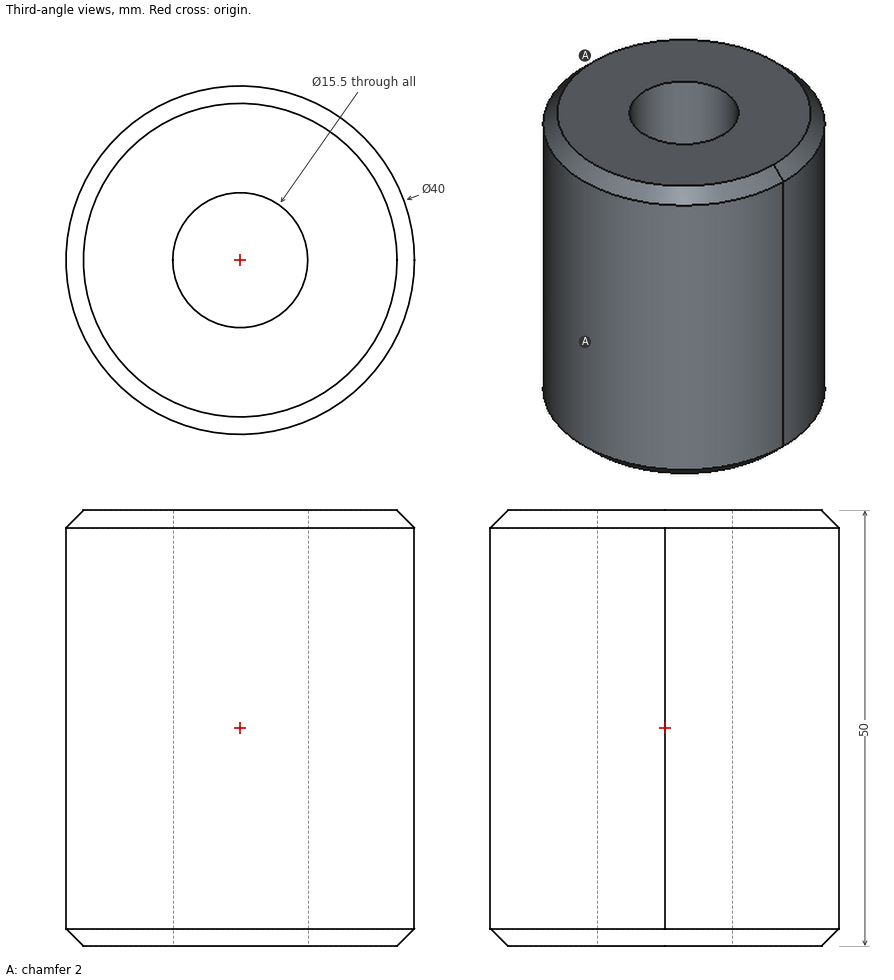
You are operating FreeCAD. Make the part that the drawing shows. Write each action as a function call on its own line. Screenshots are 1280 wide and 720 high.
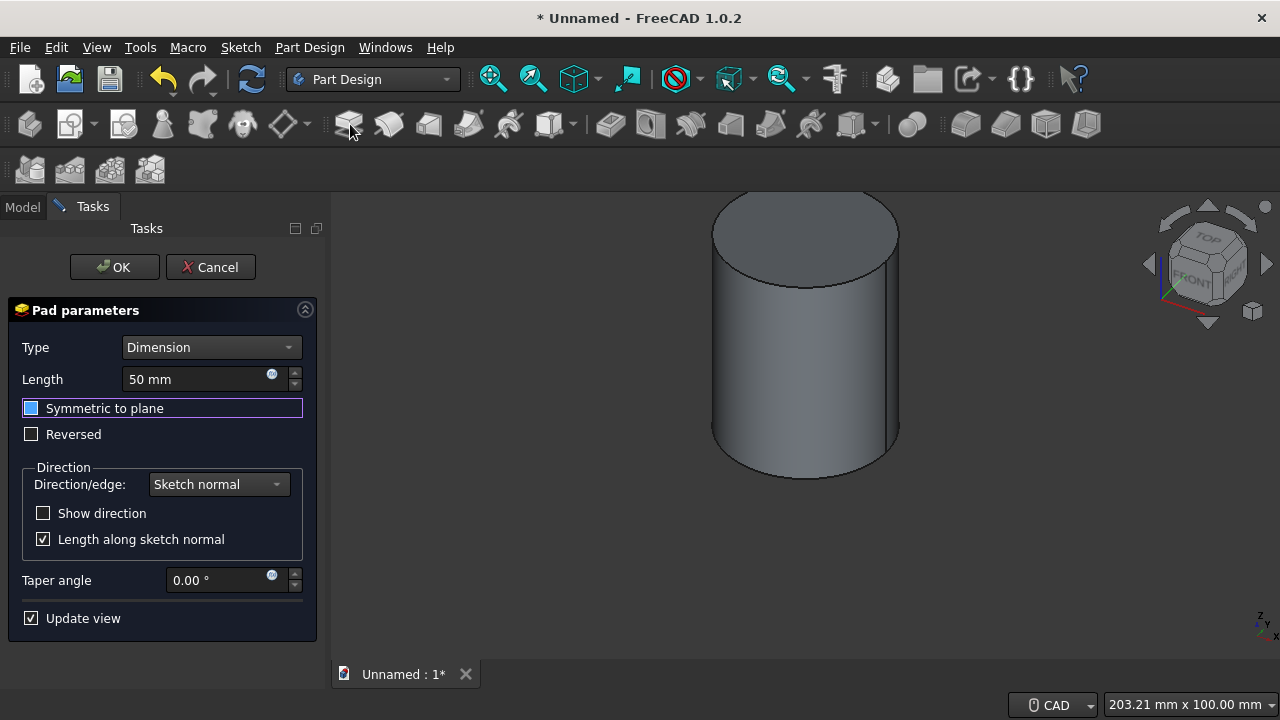
click(30, 408)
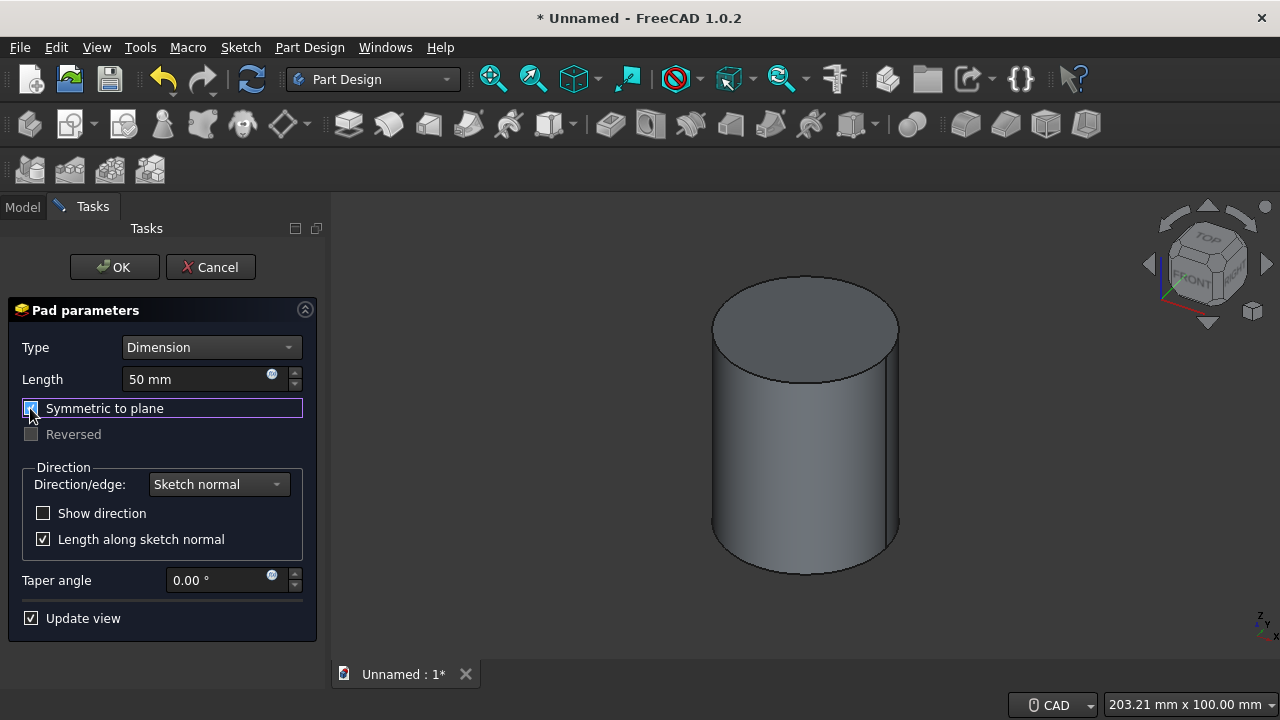
click(115, 267)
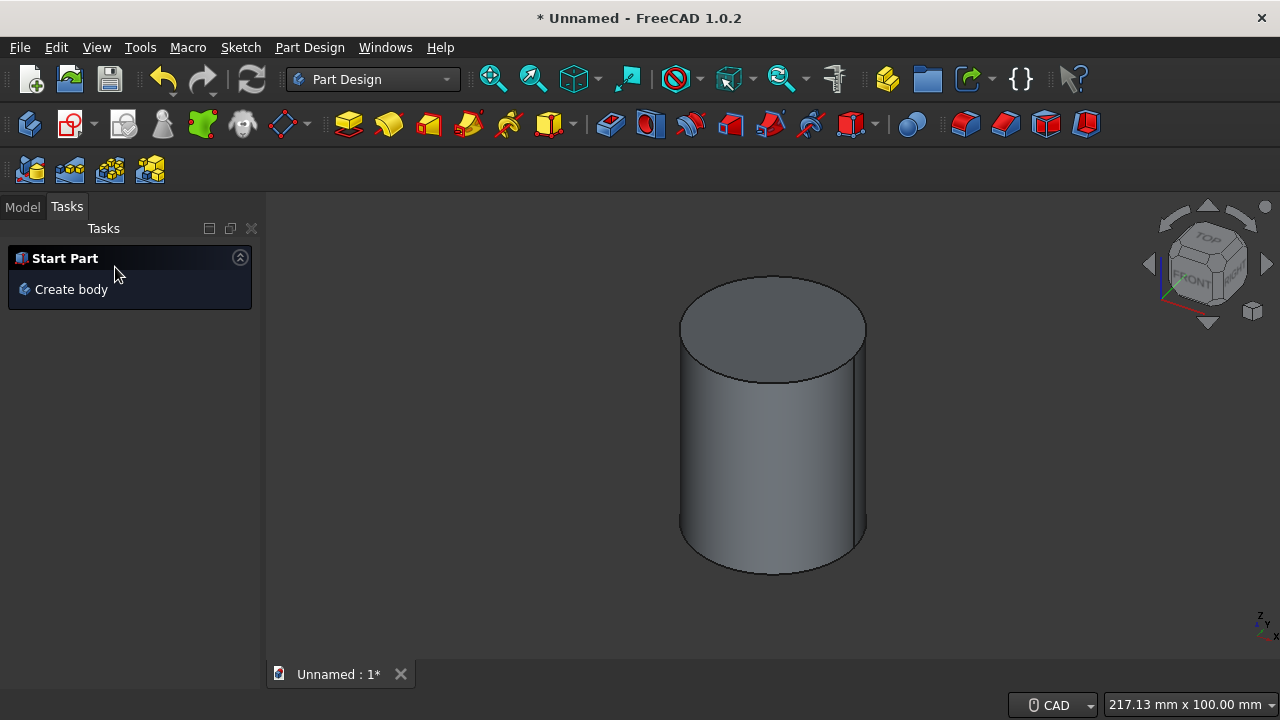
click(680, 334)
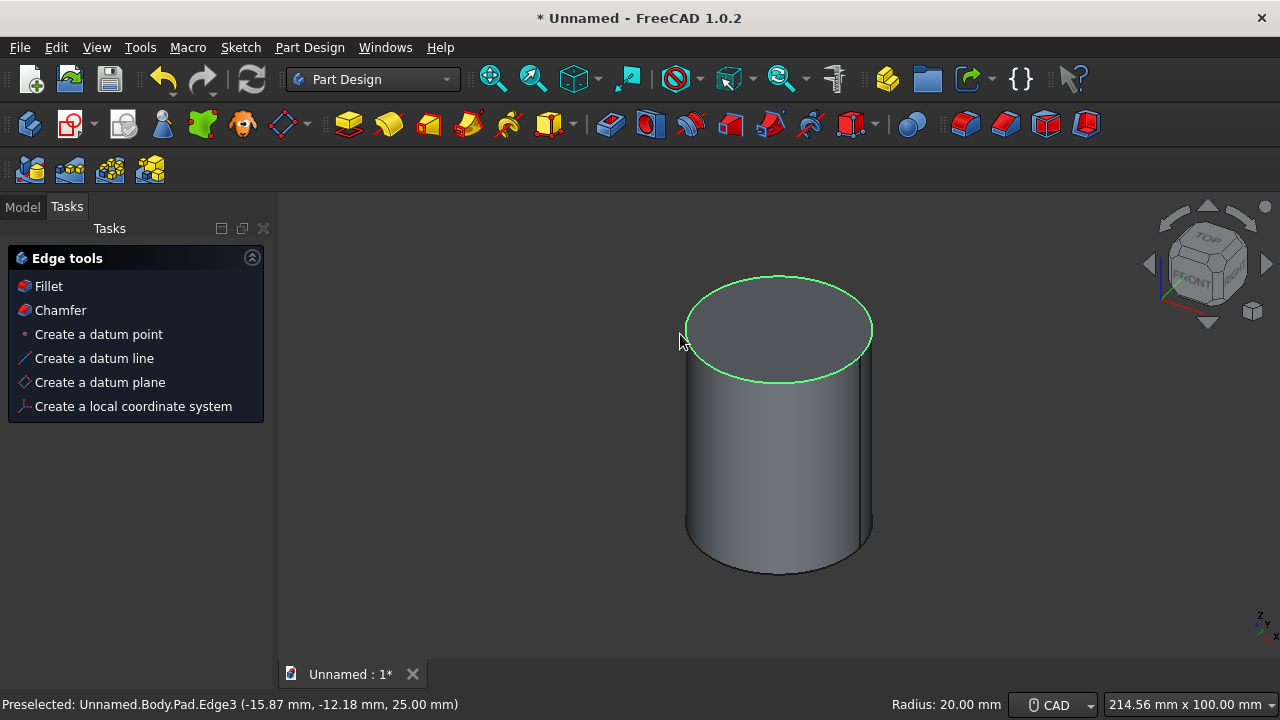
key(0)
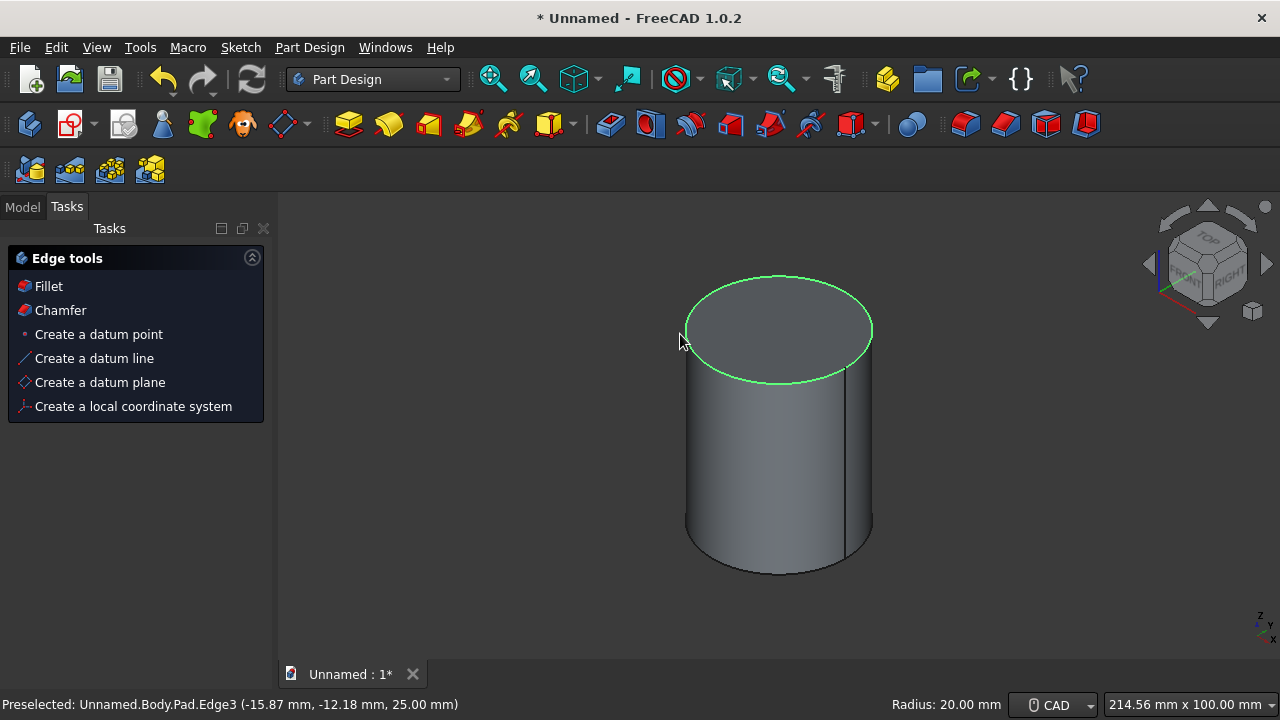
key(2)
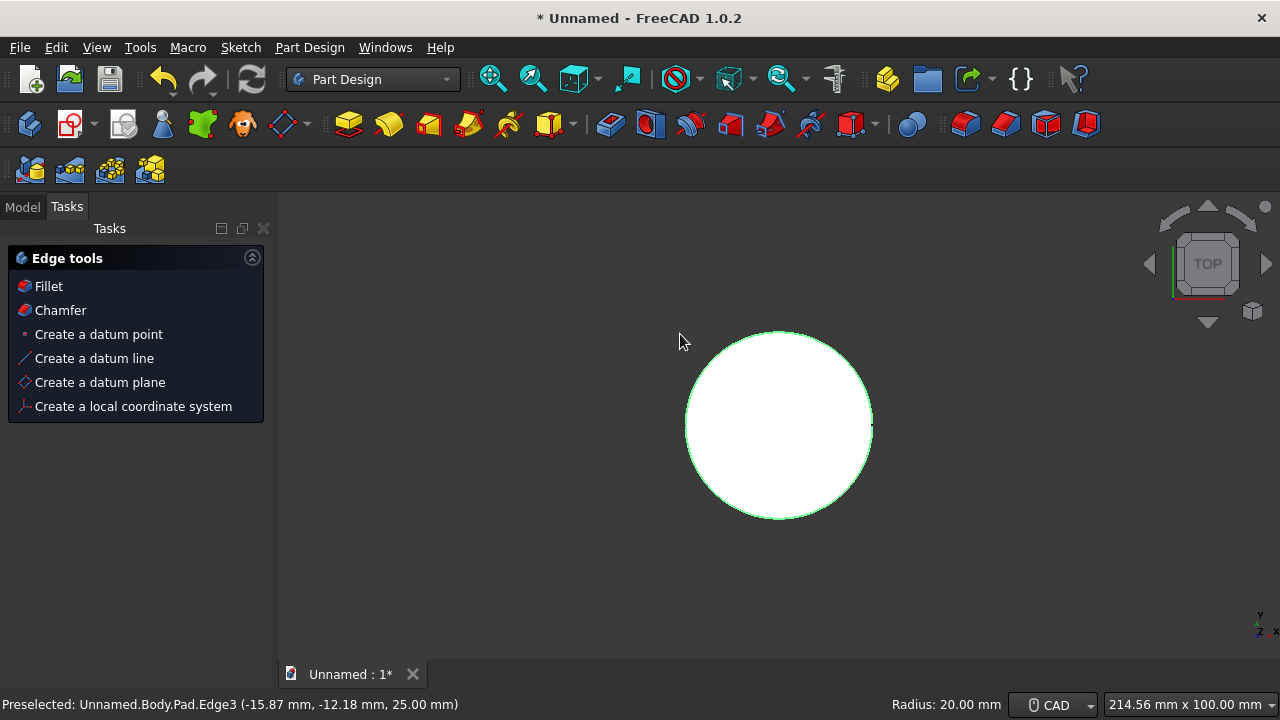
key(v)
key(f)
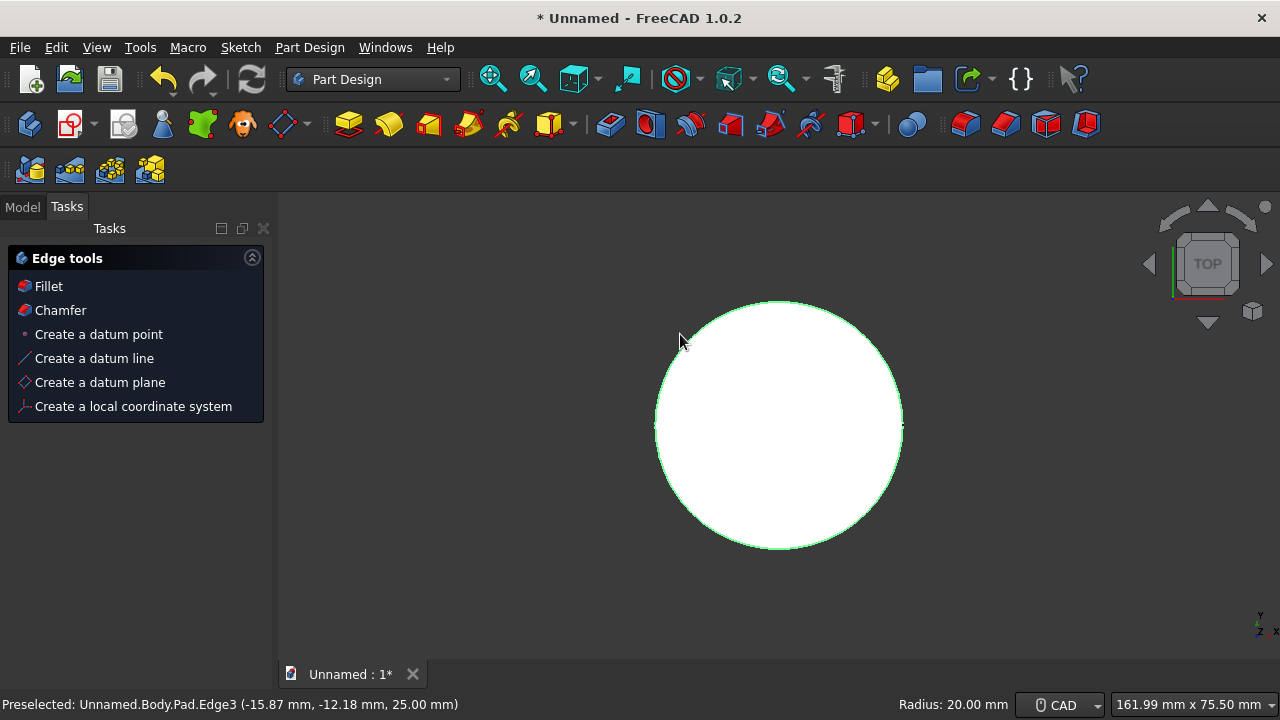
key(1)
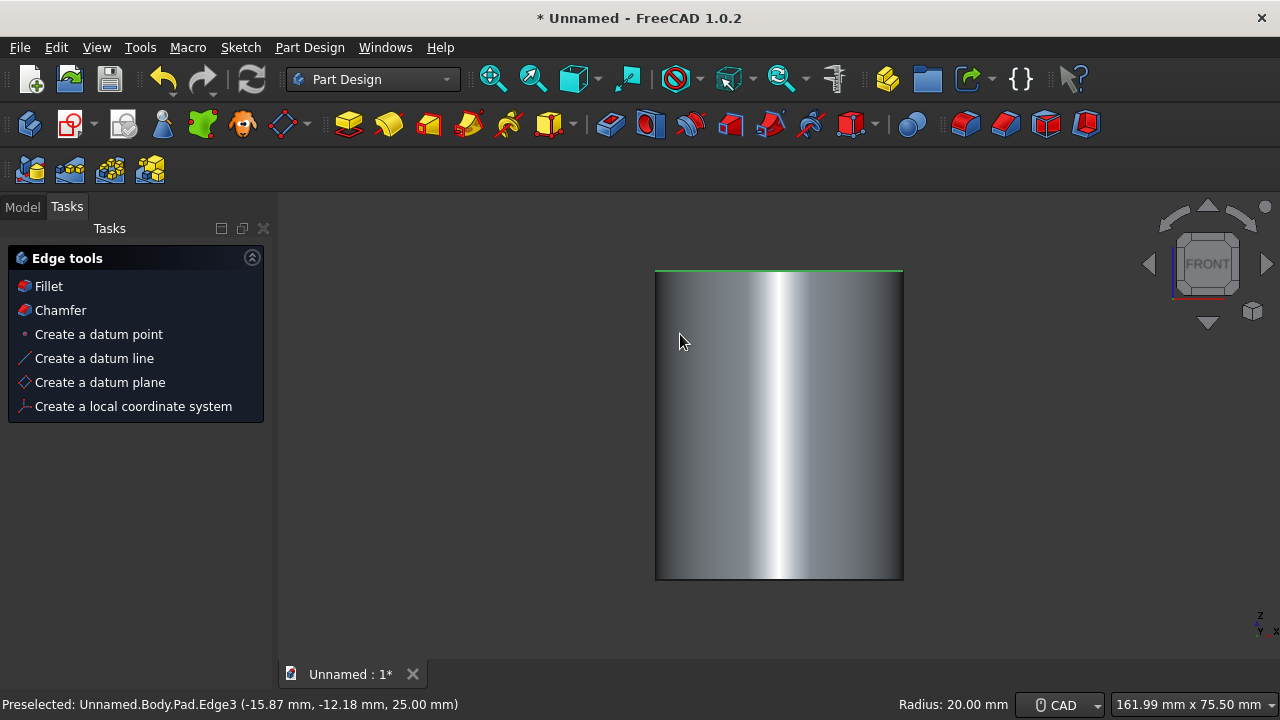
click(679, 579, ctrl)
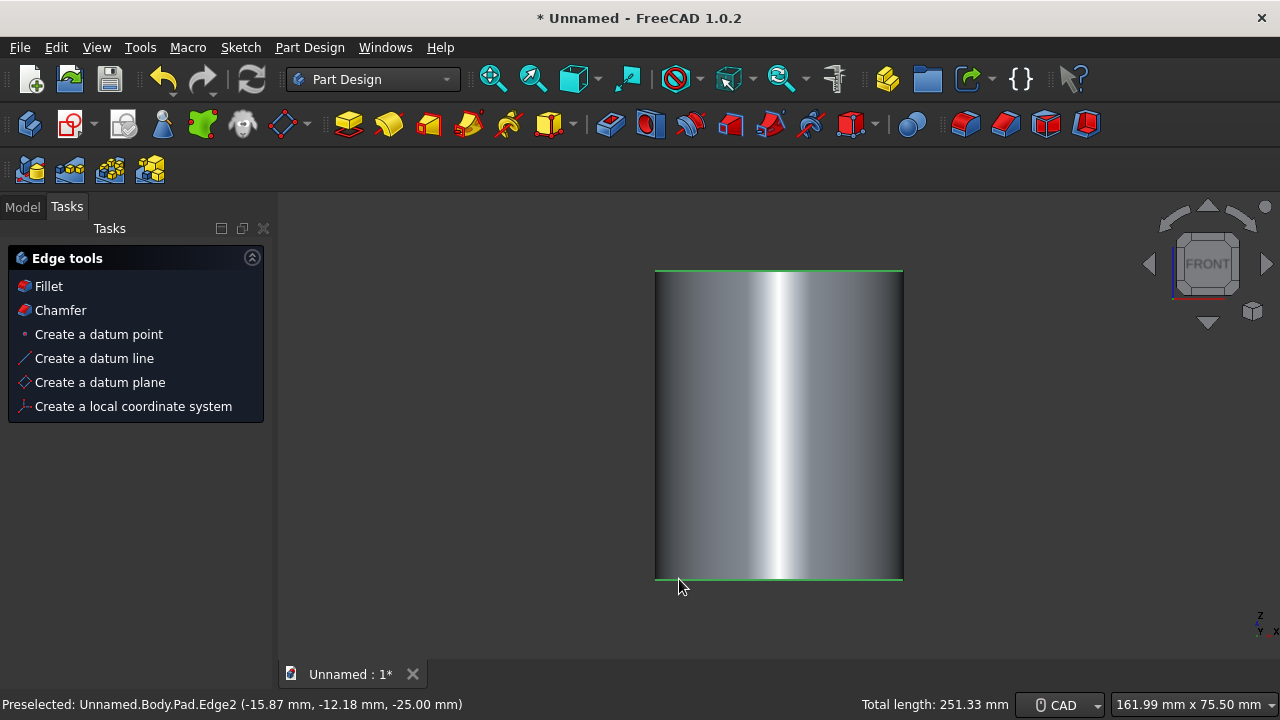
click(1006, 124)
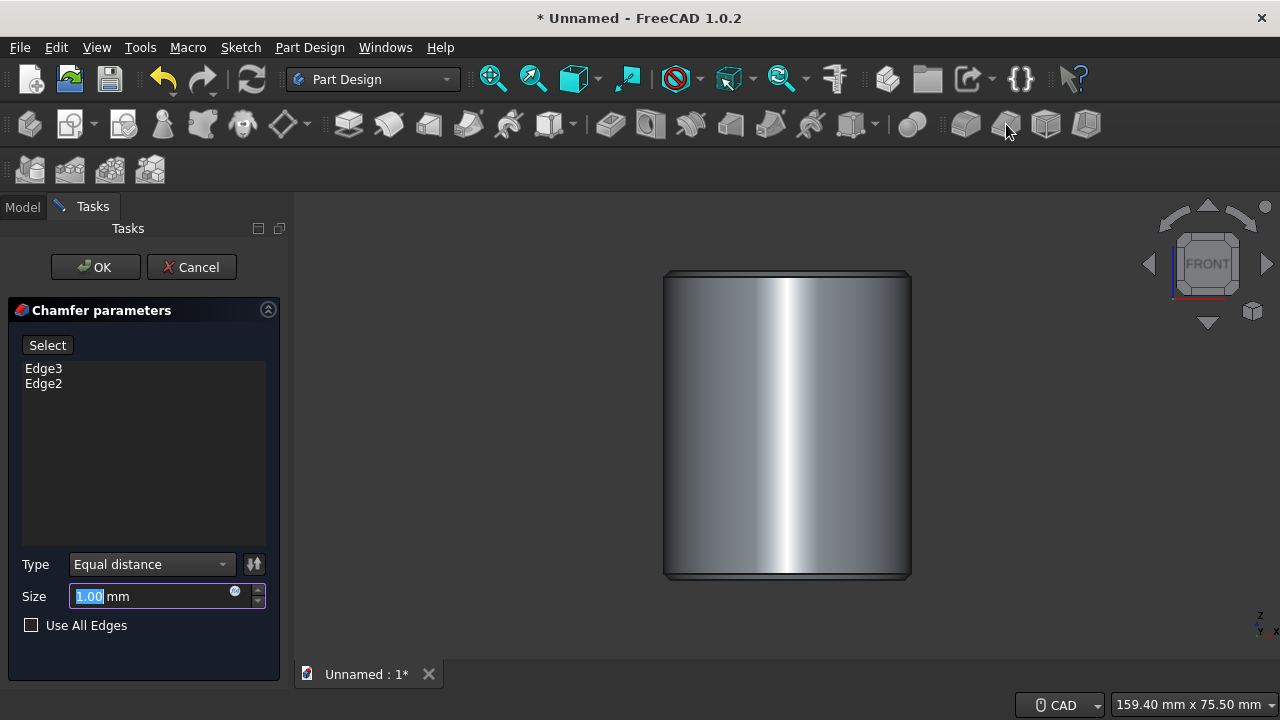
text(2)
key(Tab)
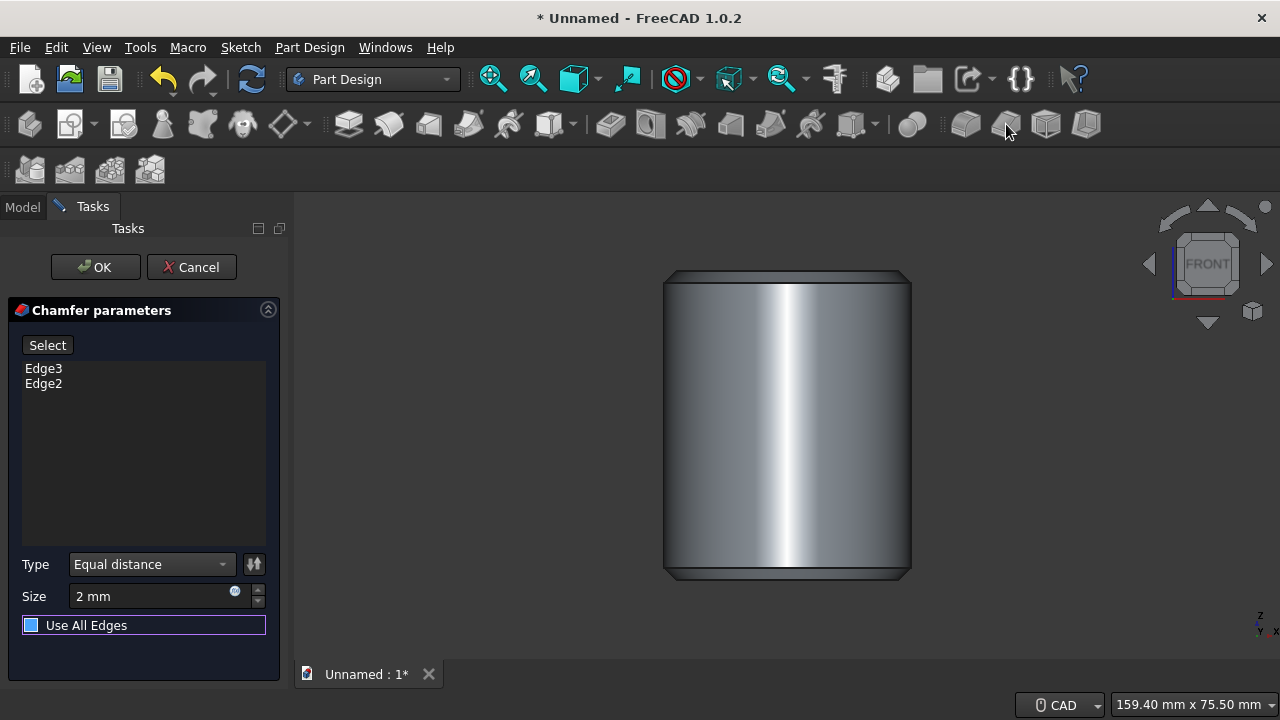
click(96, 267)